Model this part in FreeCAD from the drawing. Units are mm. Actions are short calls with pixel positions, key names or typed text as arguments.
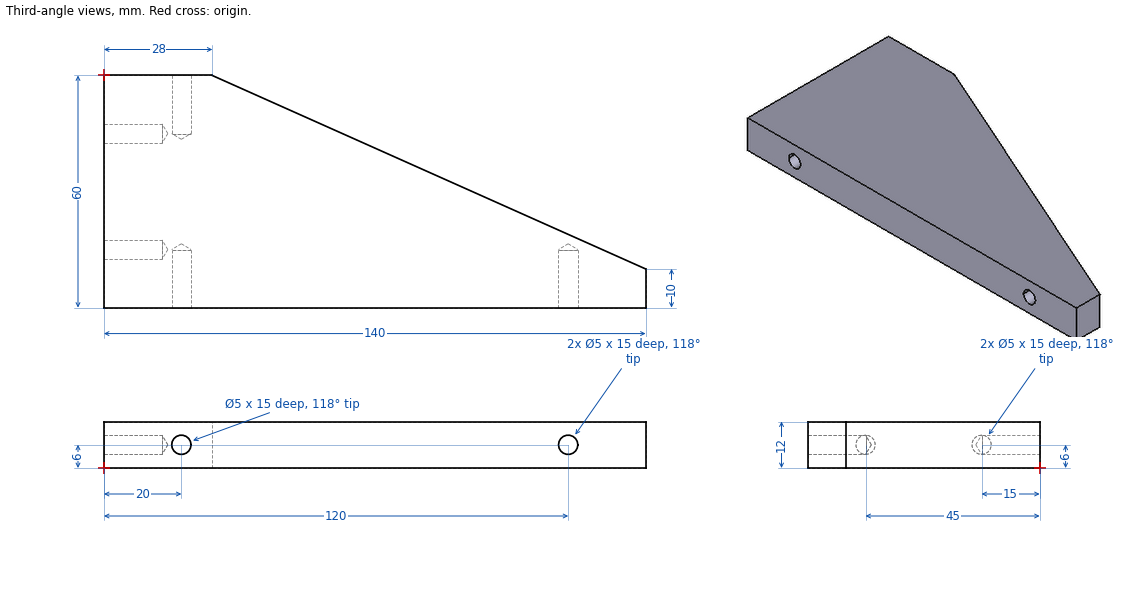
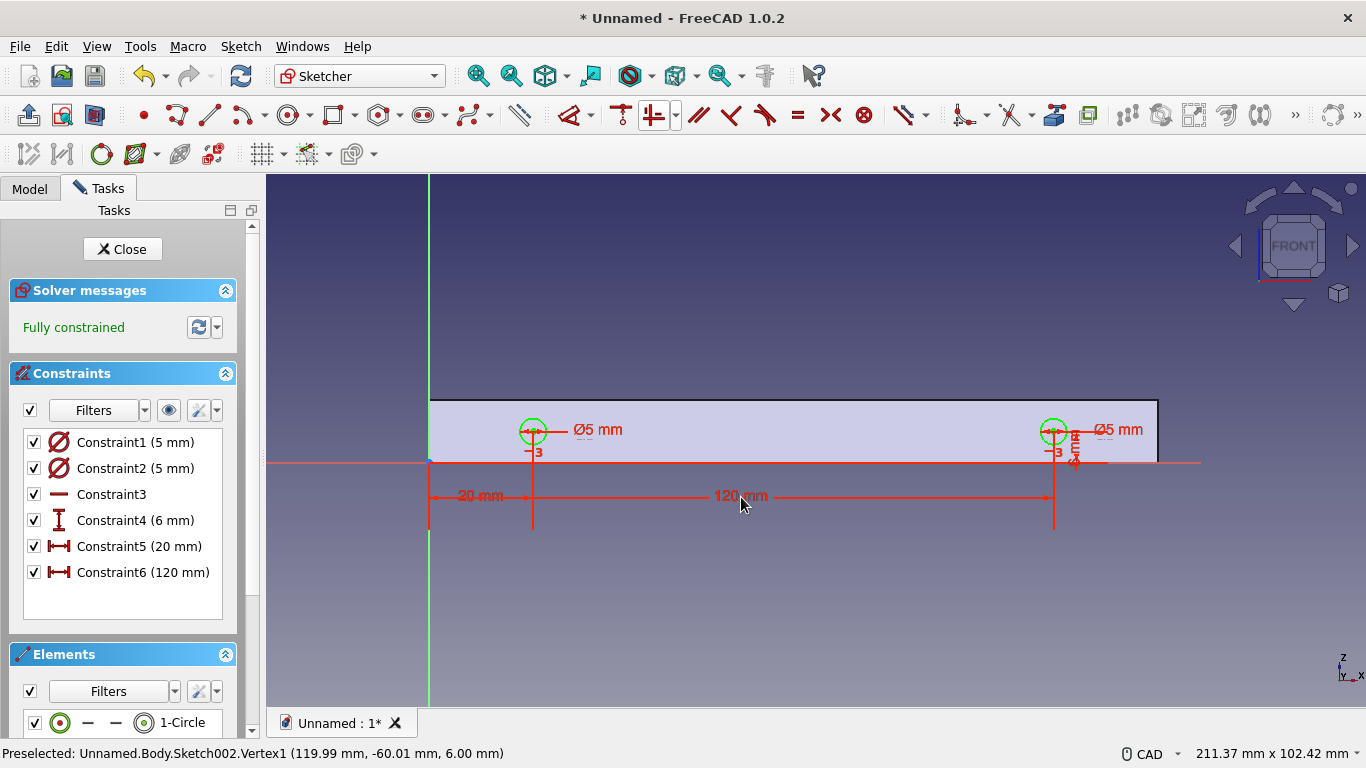
click(123, 249)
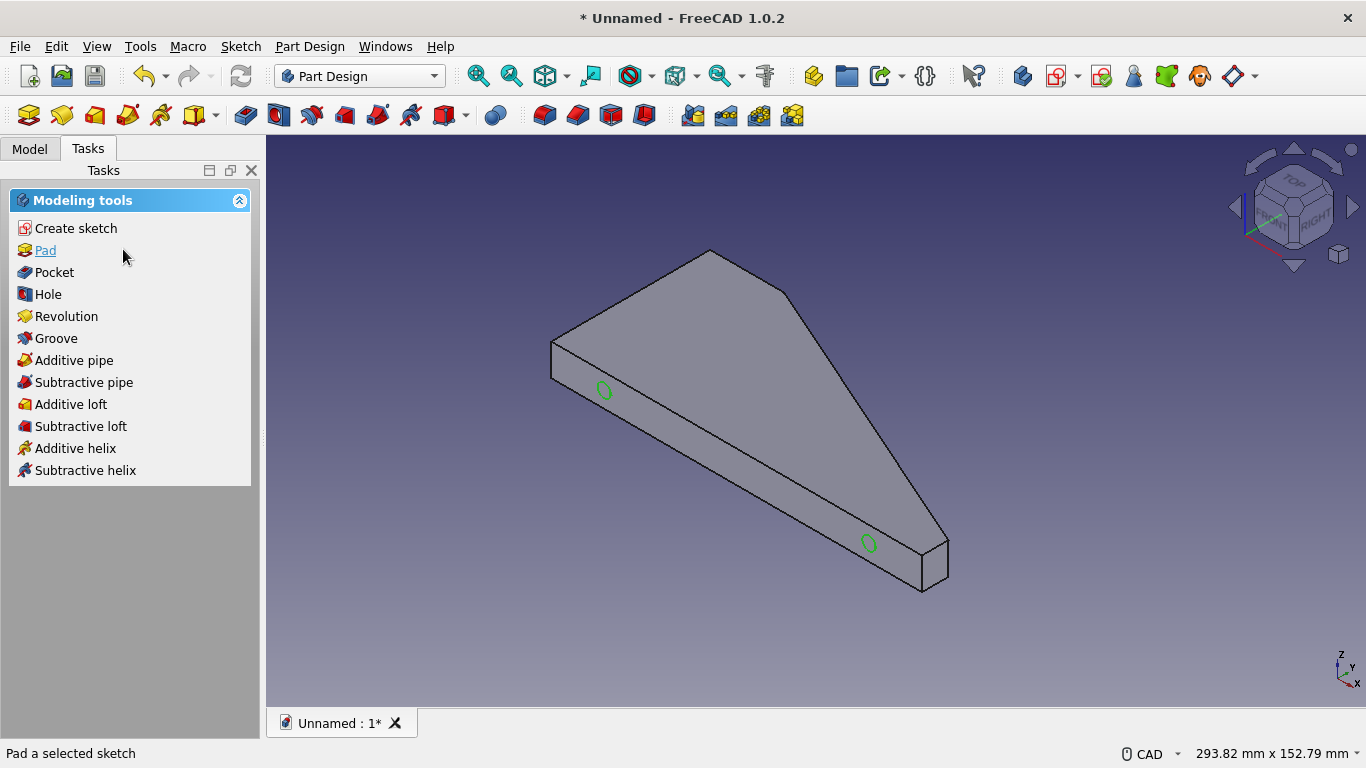
click(279, 116)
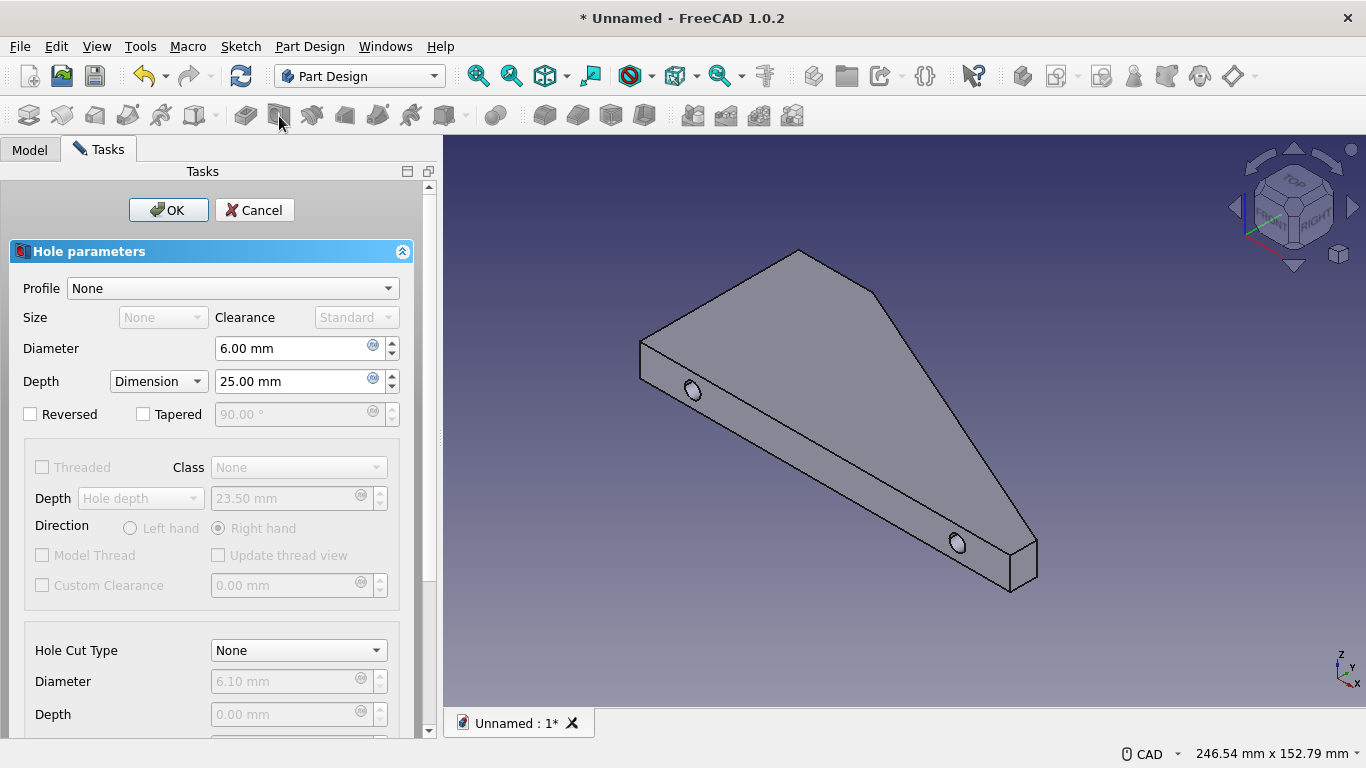
triple_click(300, 348)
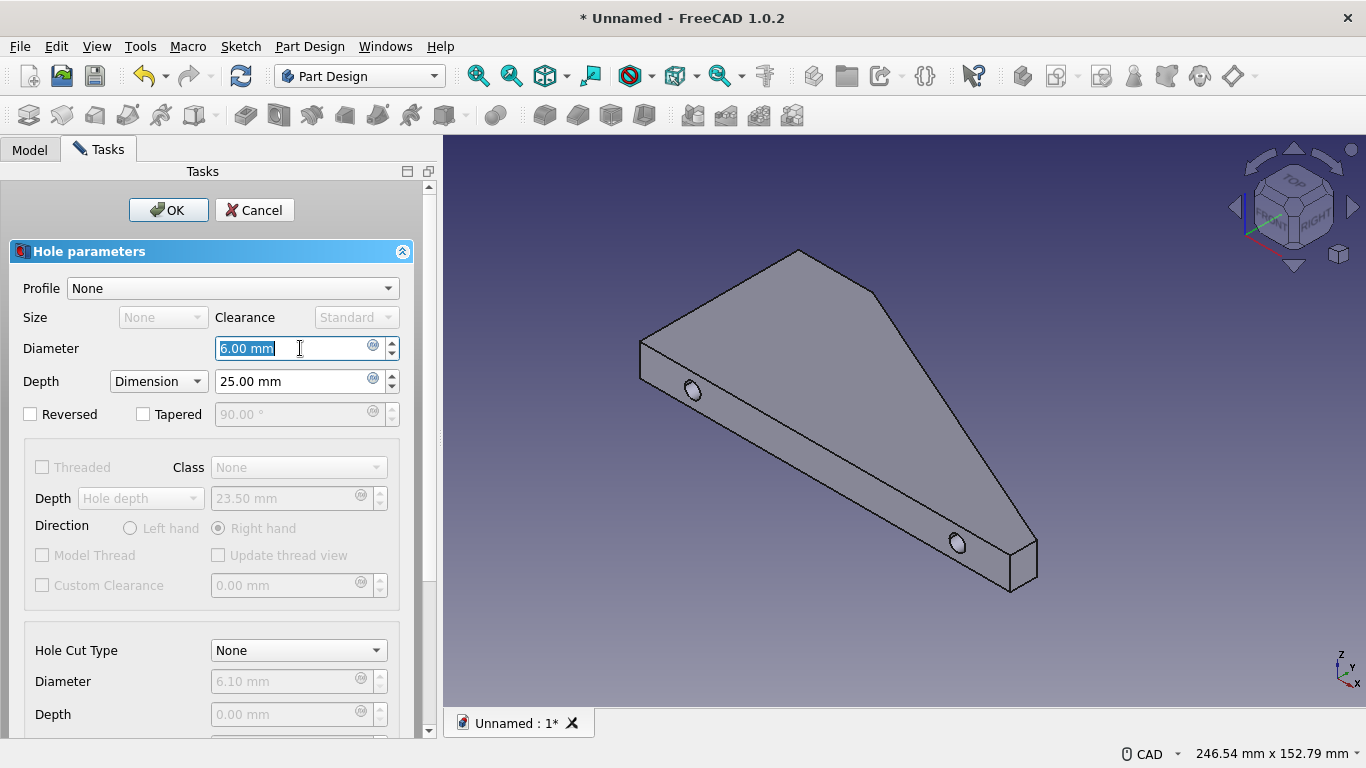
text(5)
key(Tab)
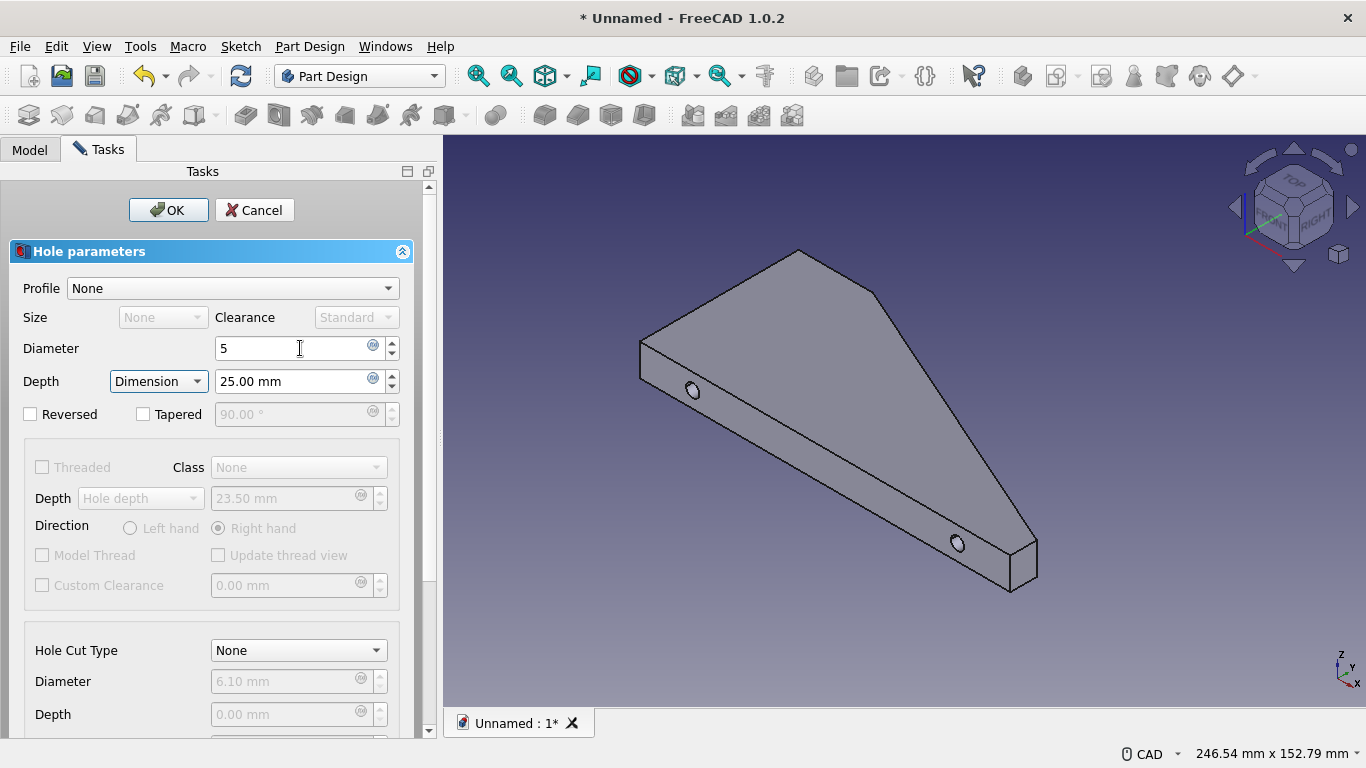
triple_click(300, 382)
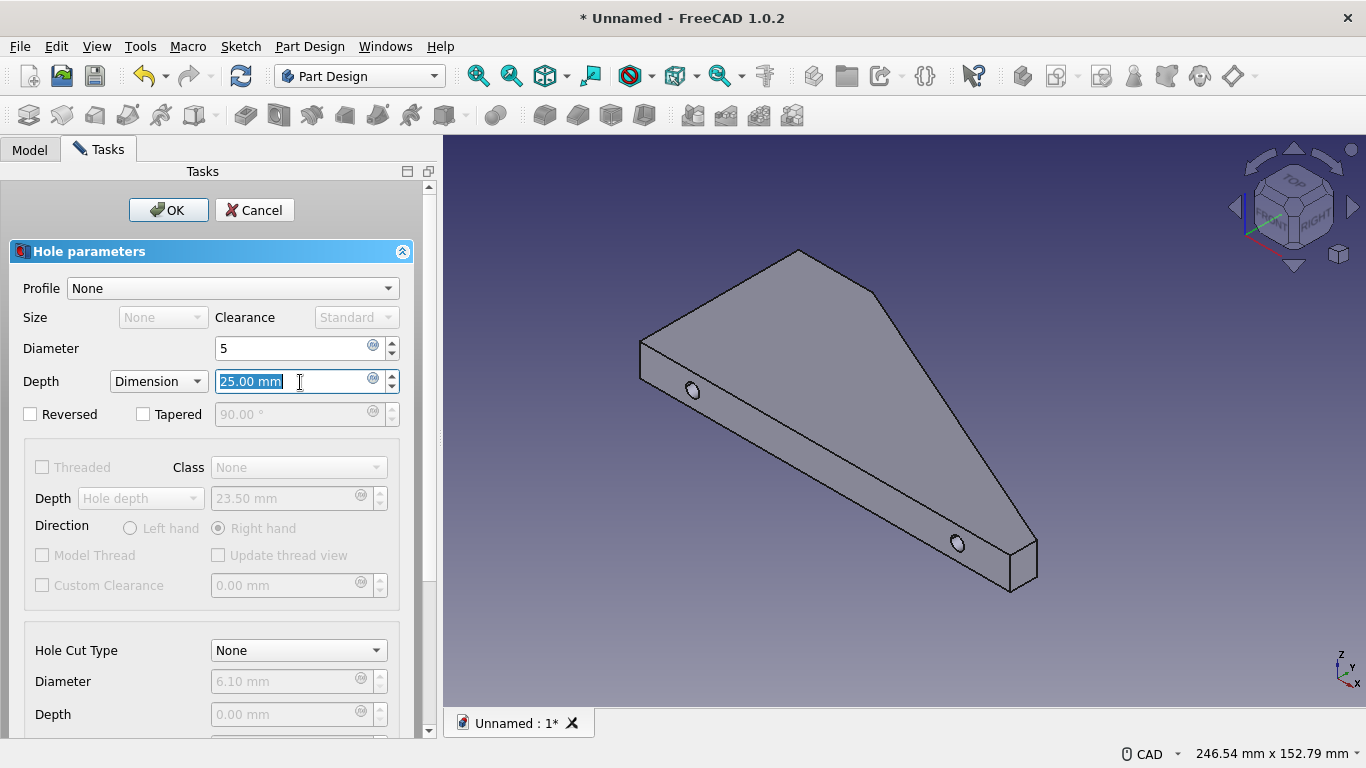
text(15)
key(Tab)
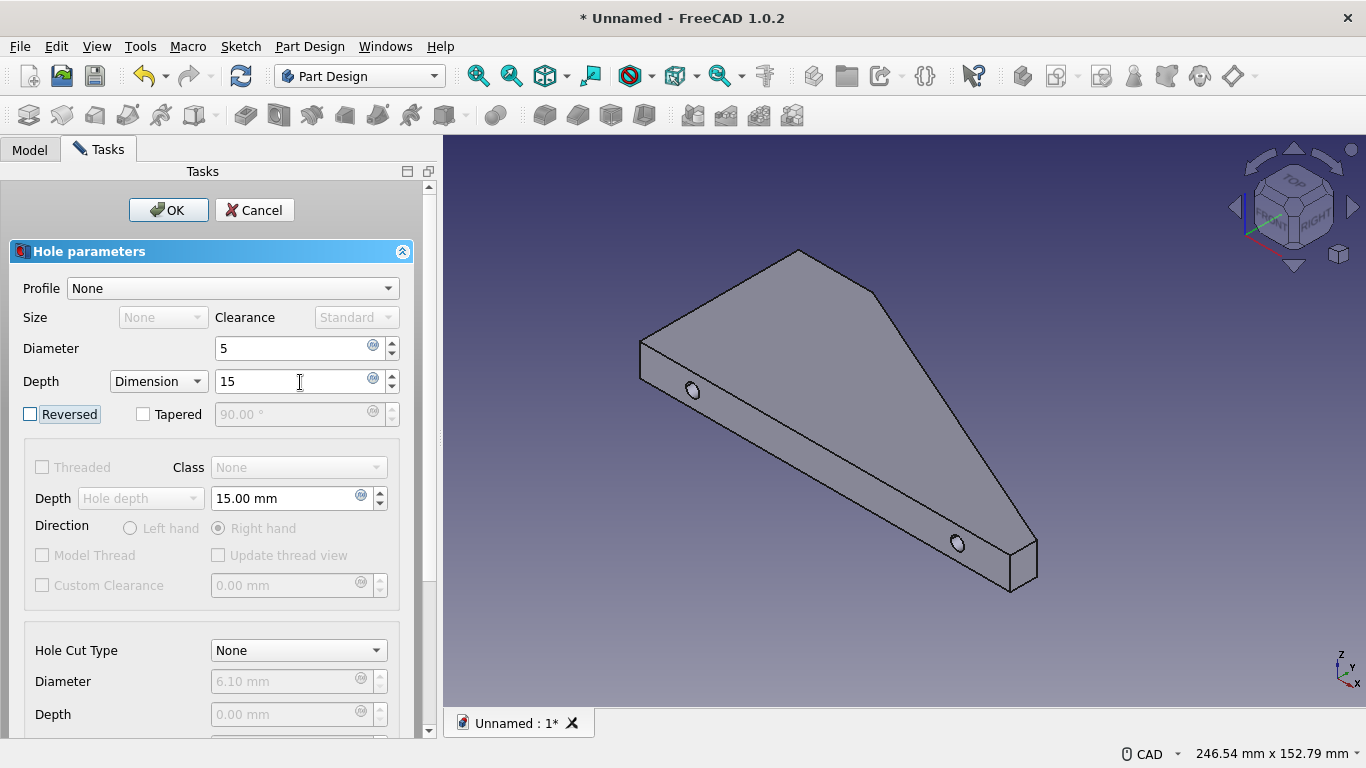
click(169, 210)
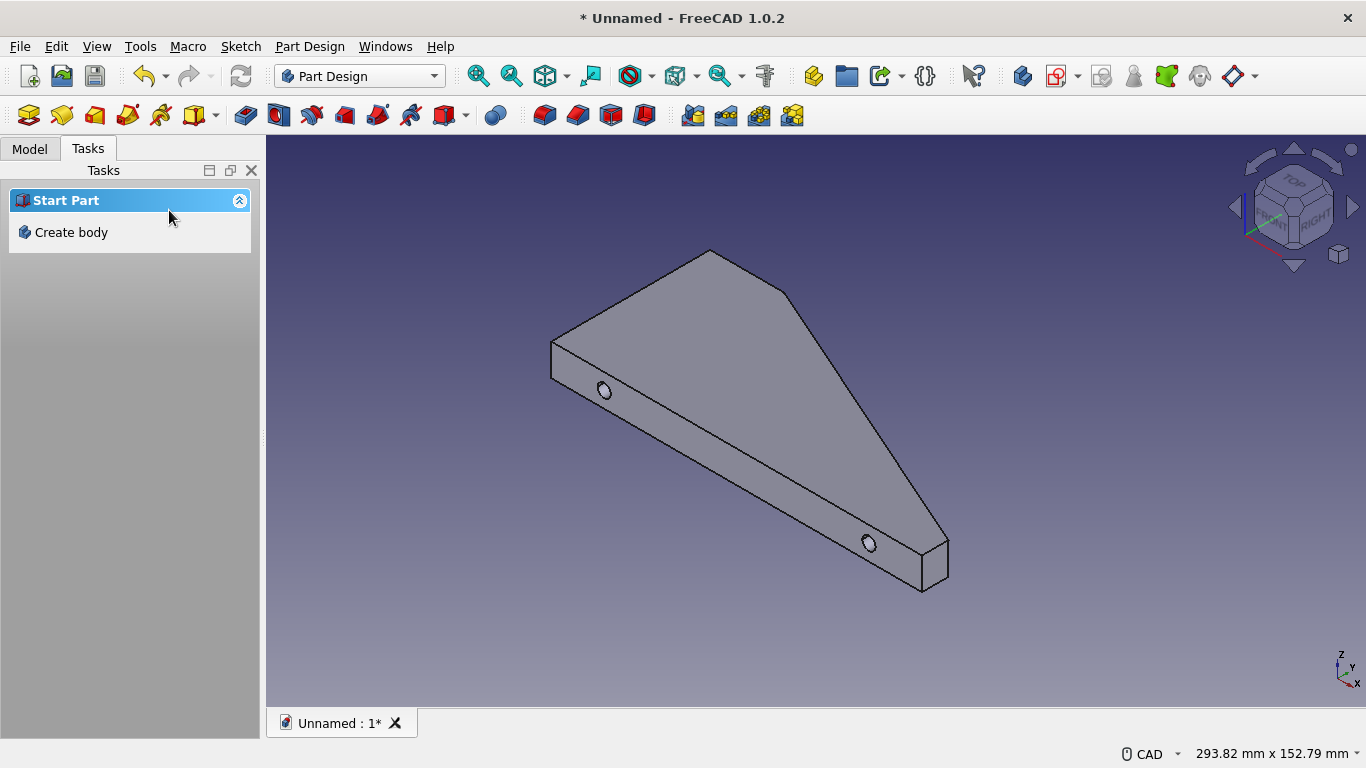
click(1056, 76)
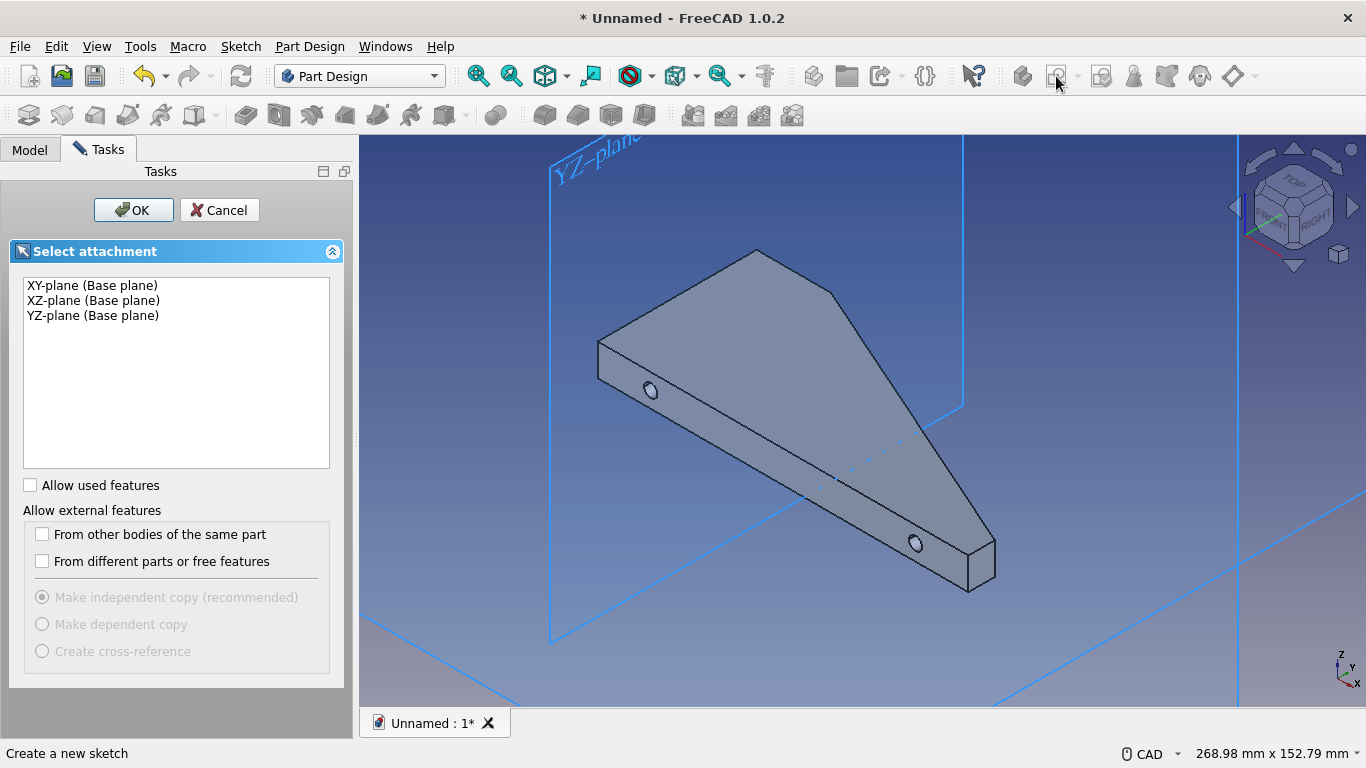
click(84, 300)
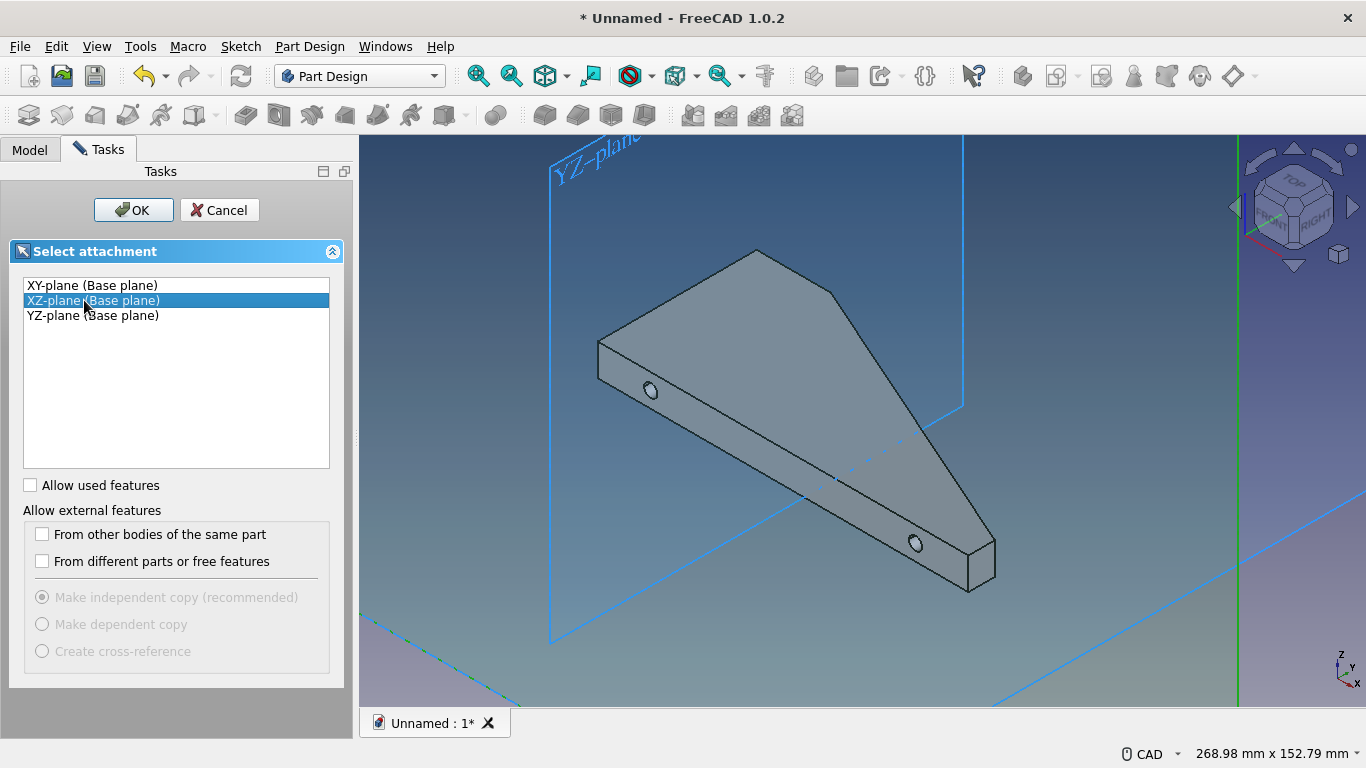
click(134, 210)